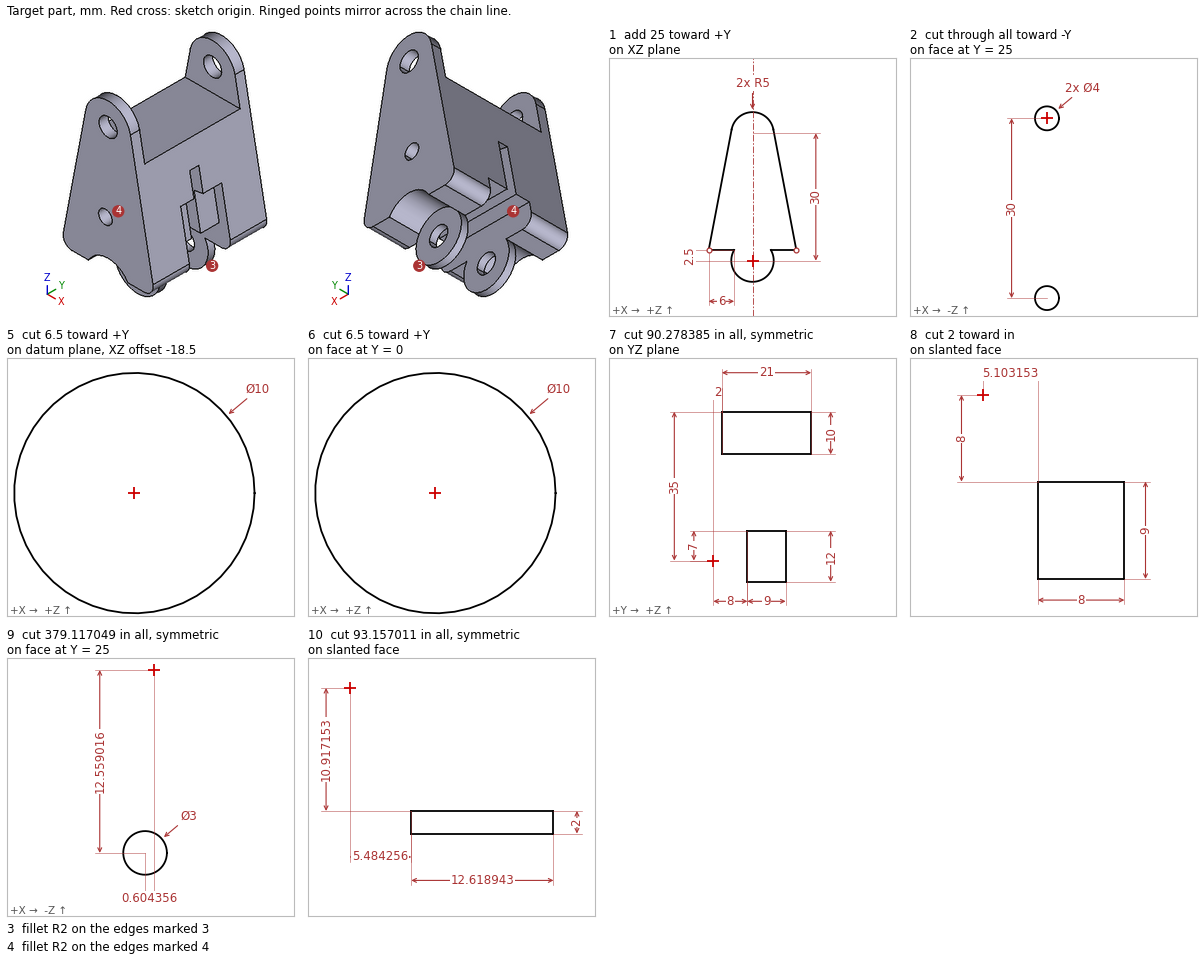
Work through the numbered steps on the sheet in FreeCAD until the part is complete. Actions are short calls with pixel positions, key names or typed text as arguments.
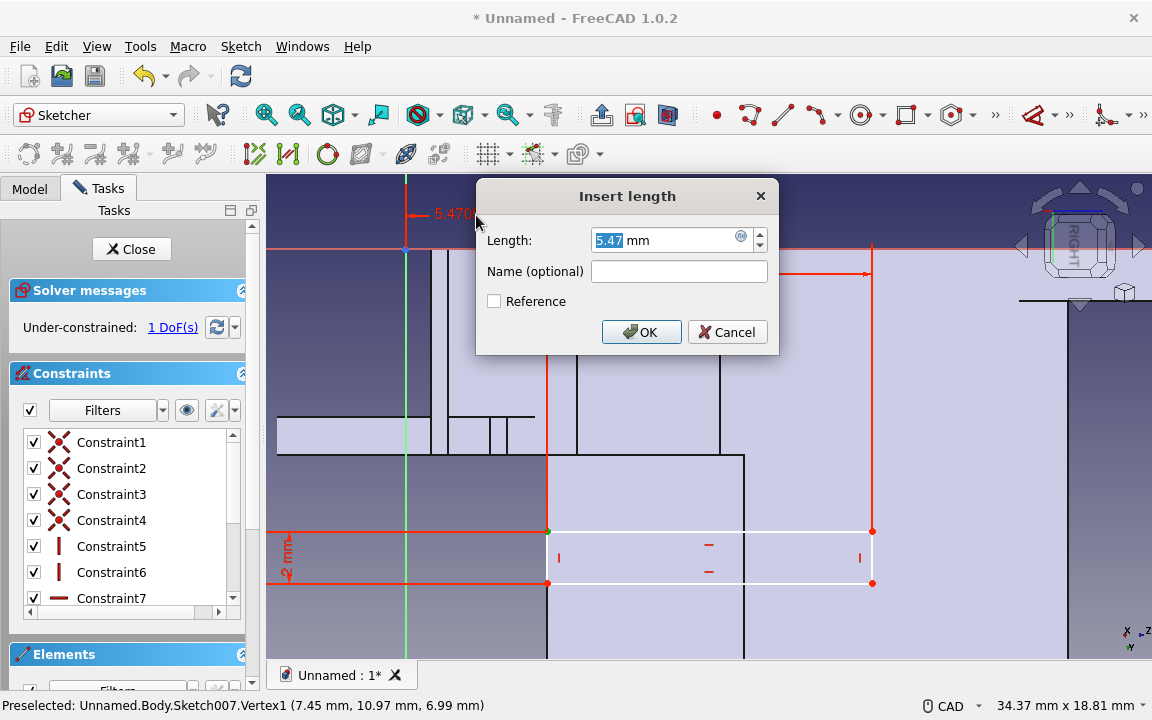
text(5.484256)
key(Return)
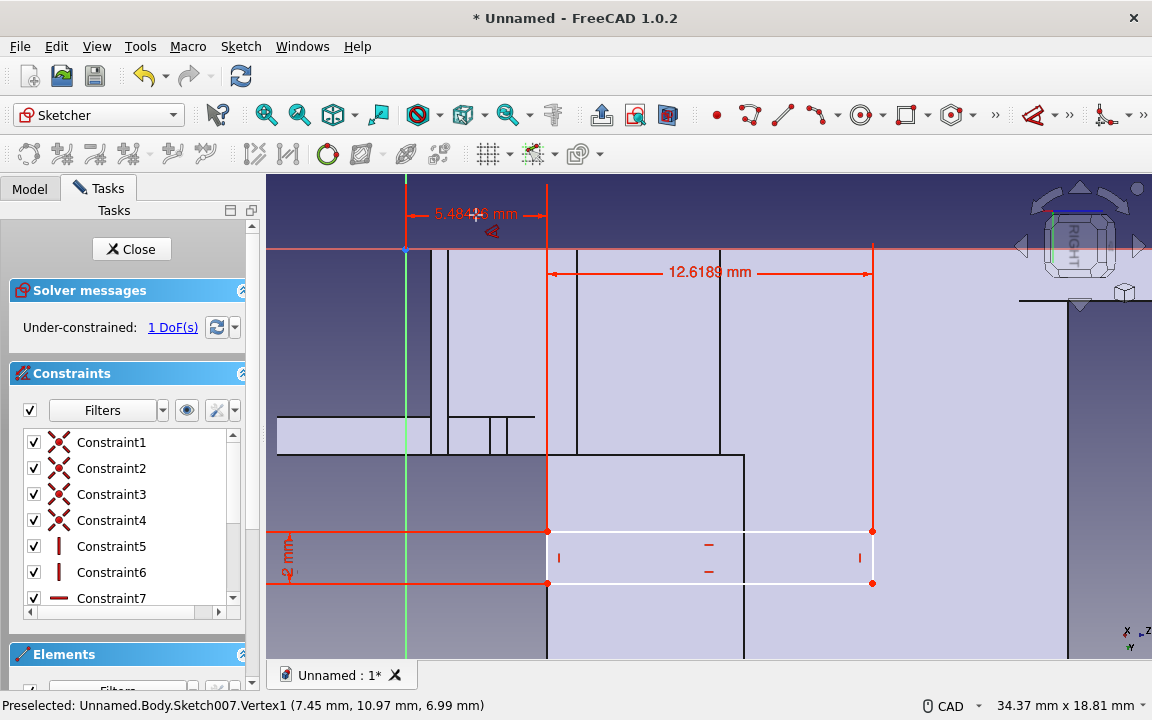
click(547, 532)
click(372, 391)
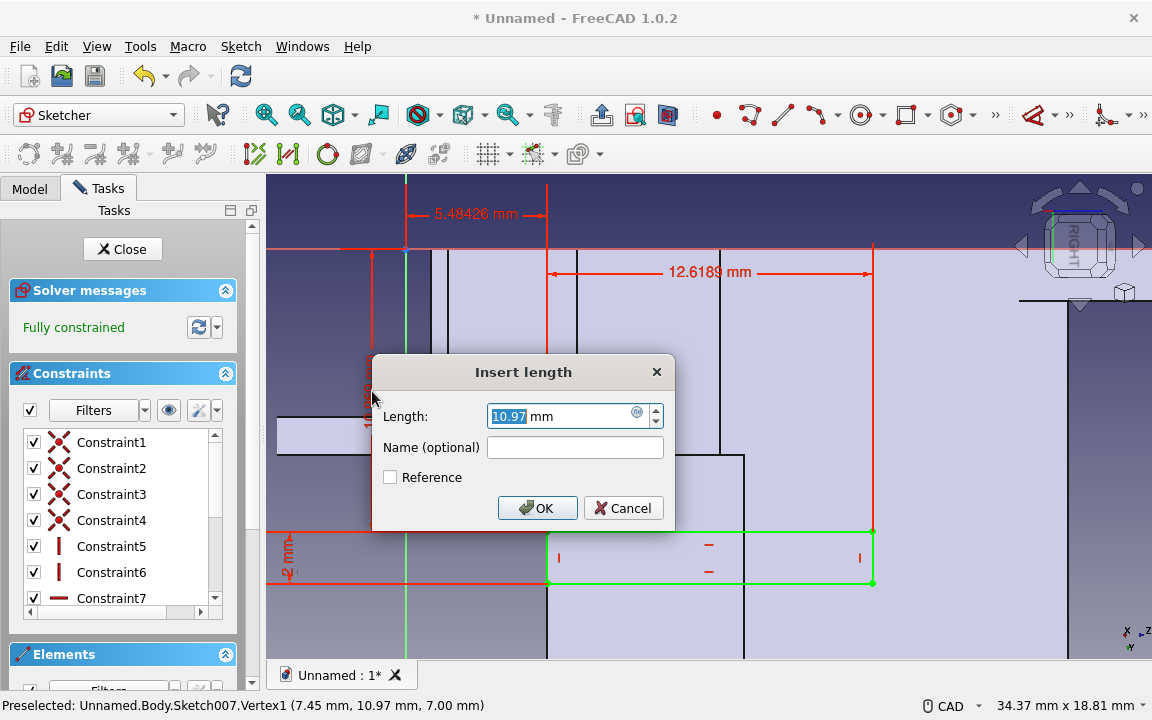
text(10.917153)
key(Return)
key(Escape)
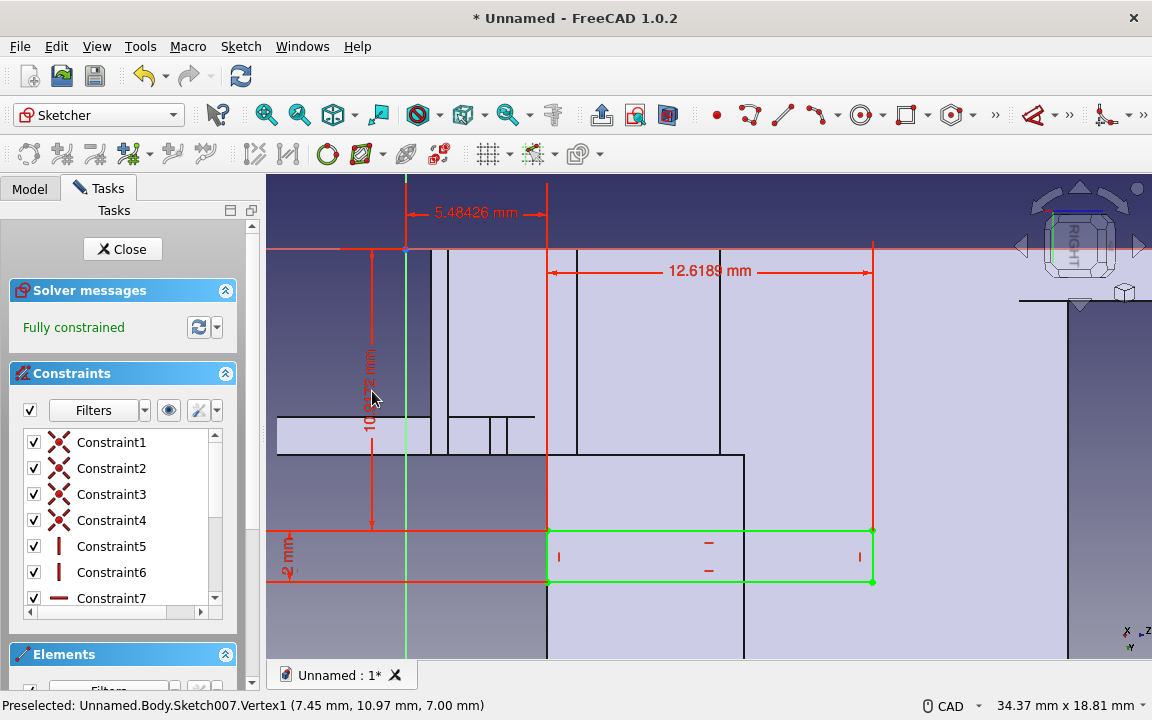
click(123, 249)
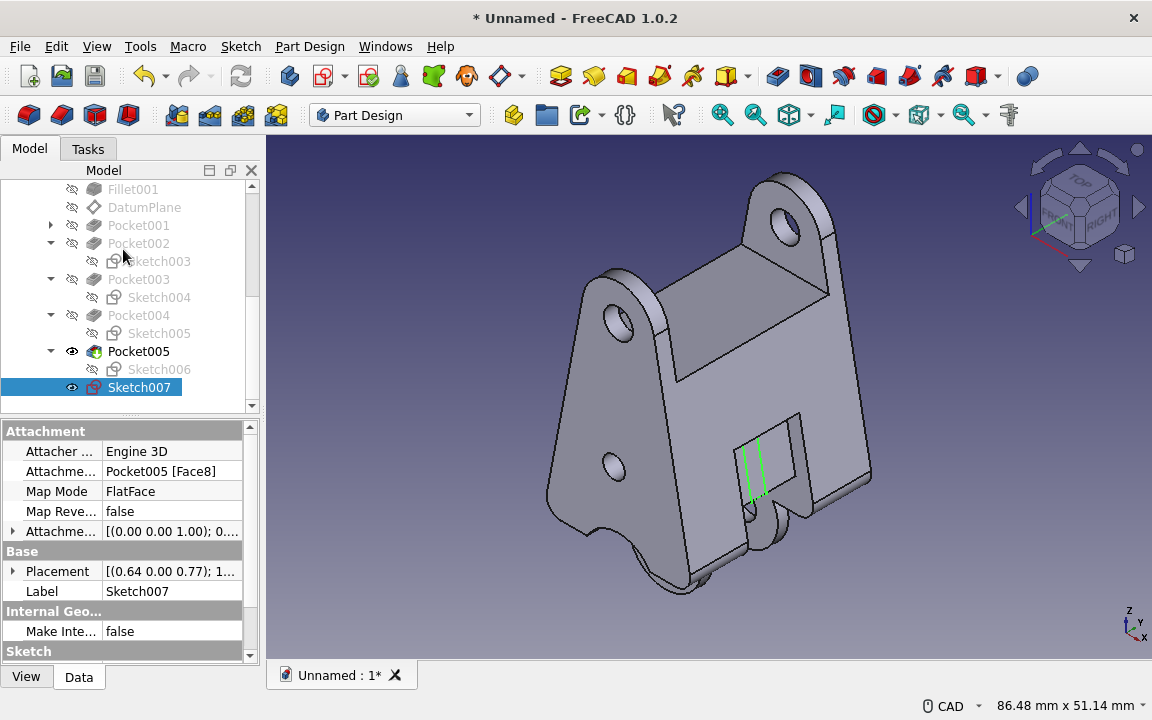
click(778, 76)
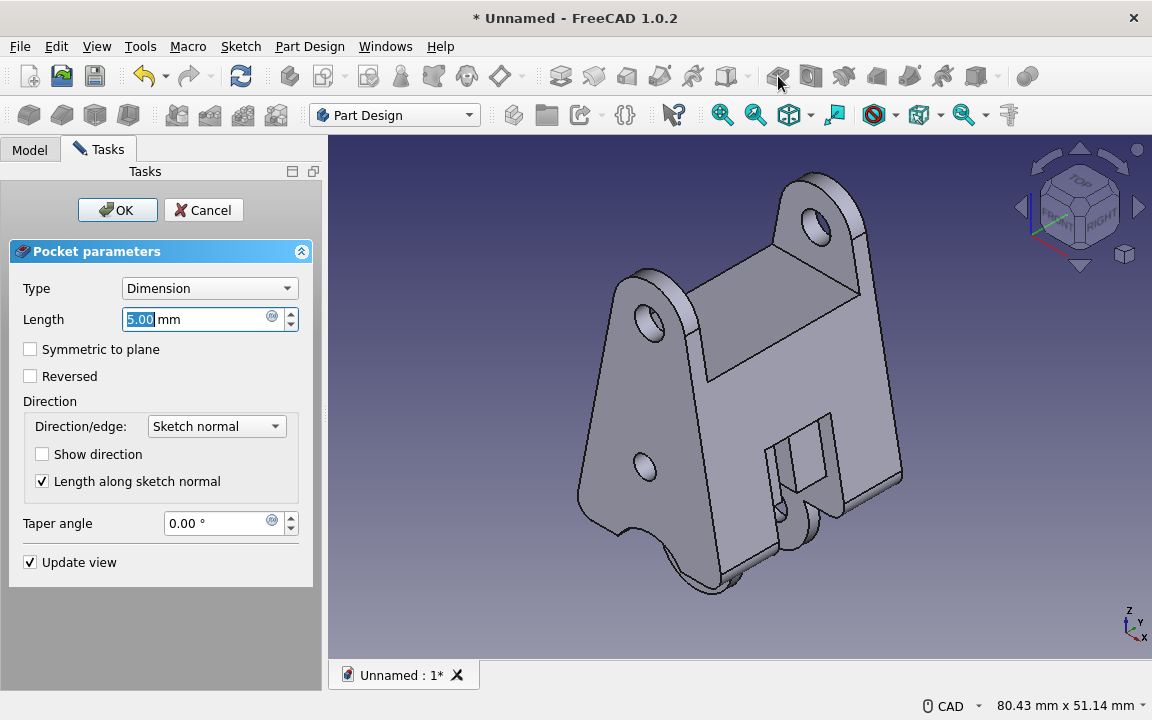
text(93.157011)
key(Tab)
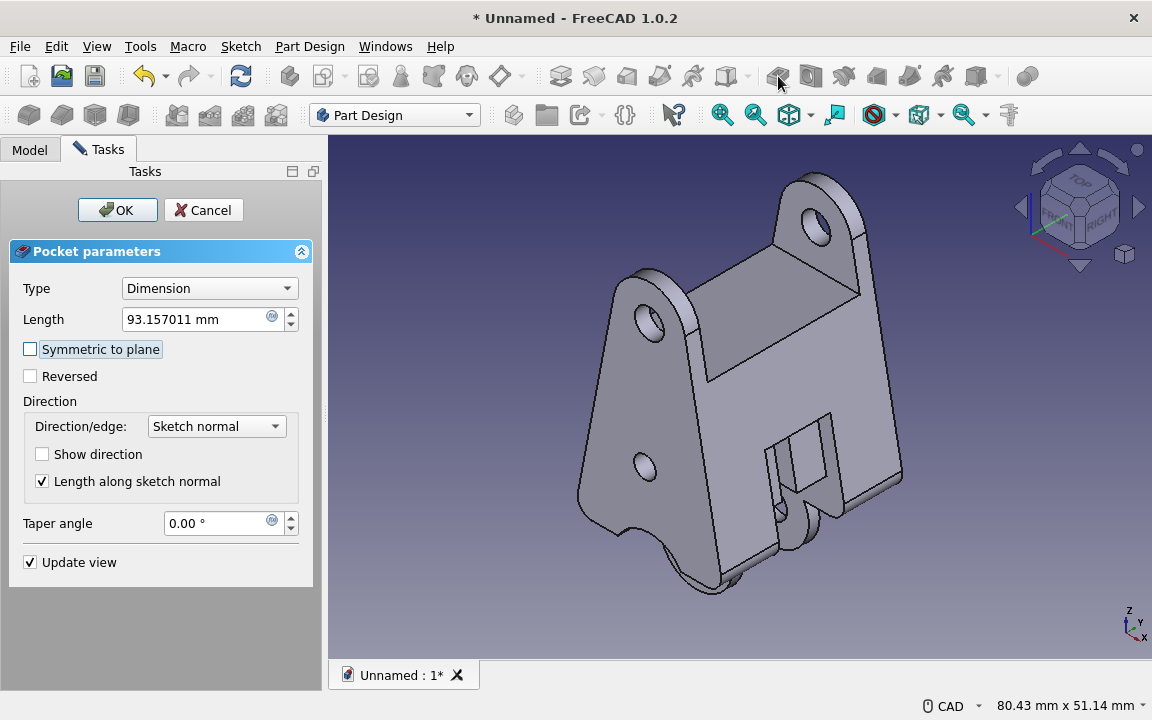
click(31, 349)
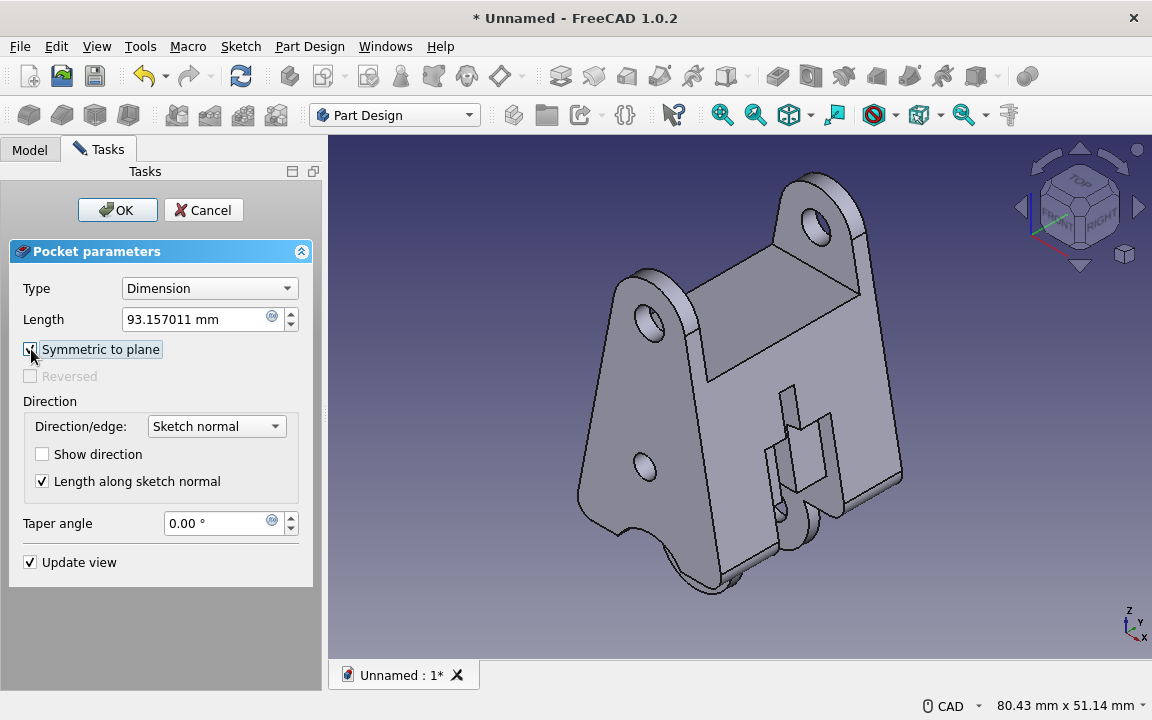
click(118, 210)